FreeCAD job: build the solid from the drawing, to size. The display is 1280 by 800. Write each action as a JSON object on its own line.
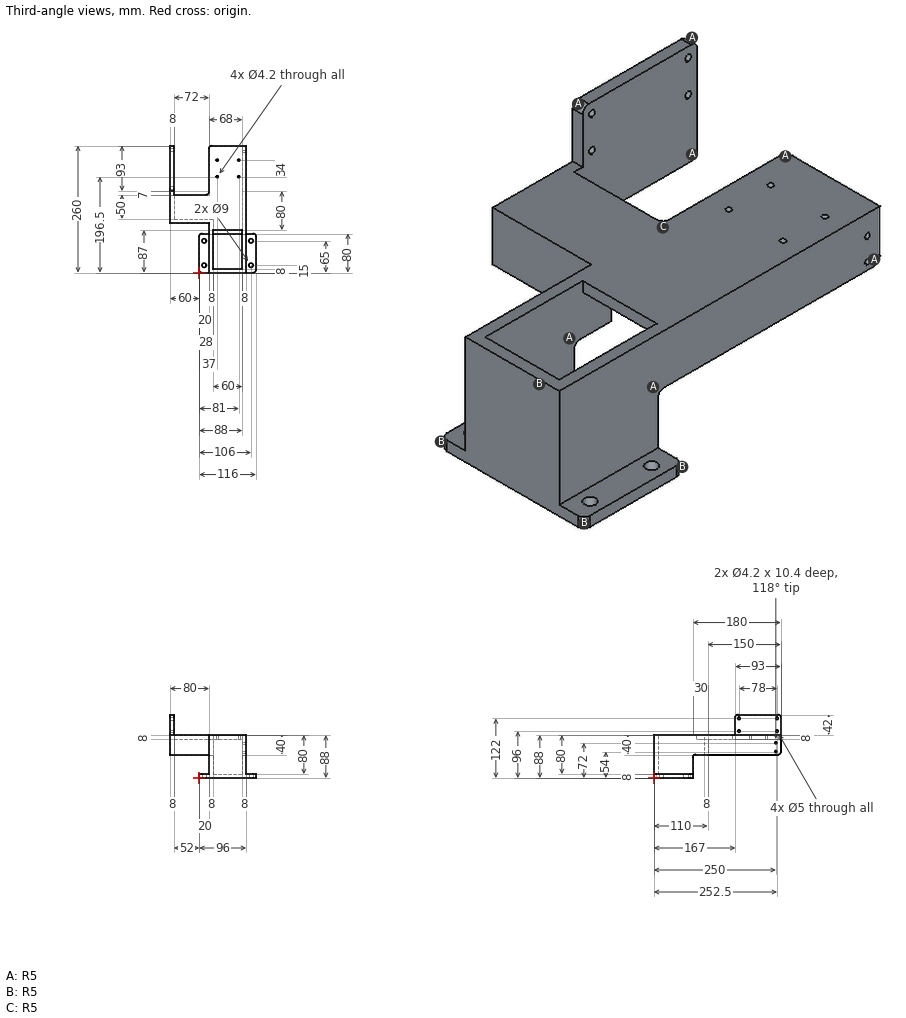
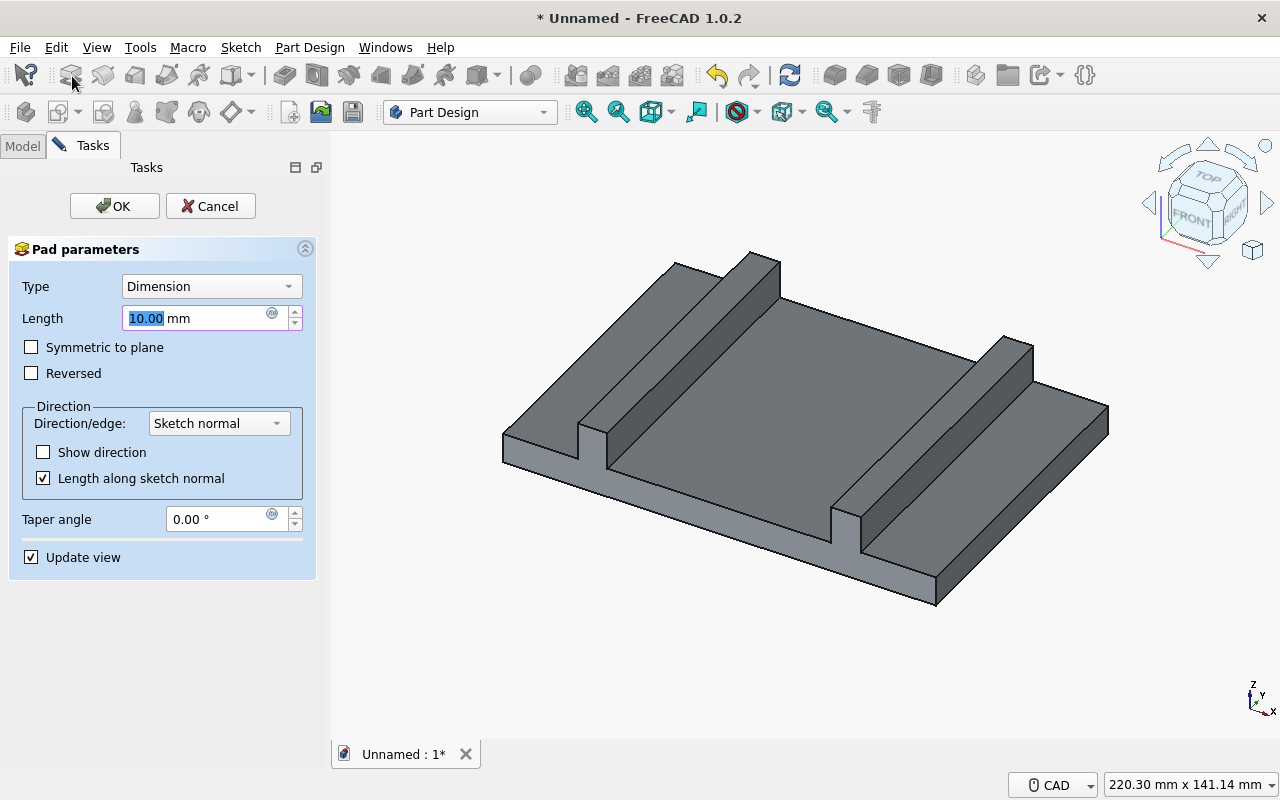
{"action": "type", "text": "80"}
{"action": "key", "text": "Tab"}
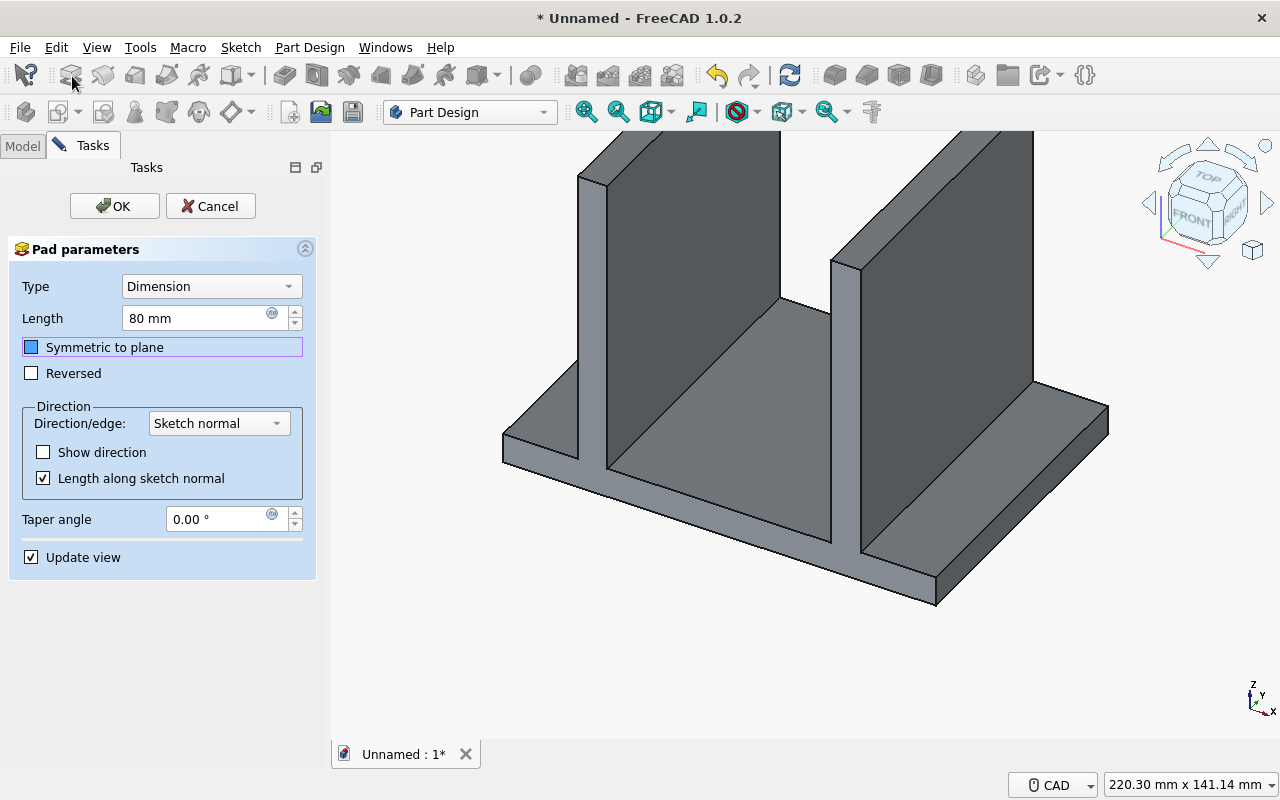
{"action": "left_click", "coordinate": [115, 206]}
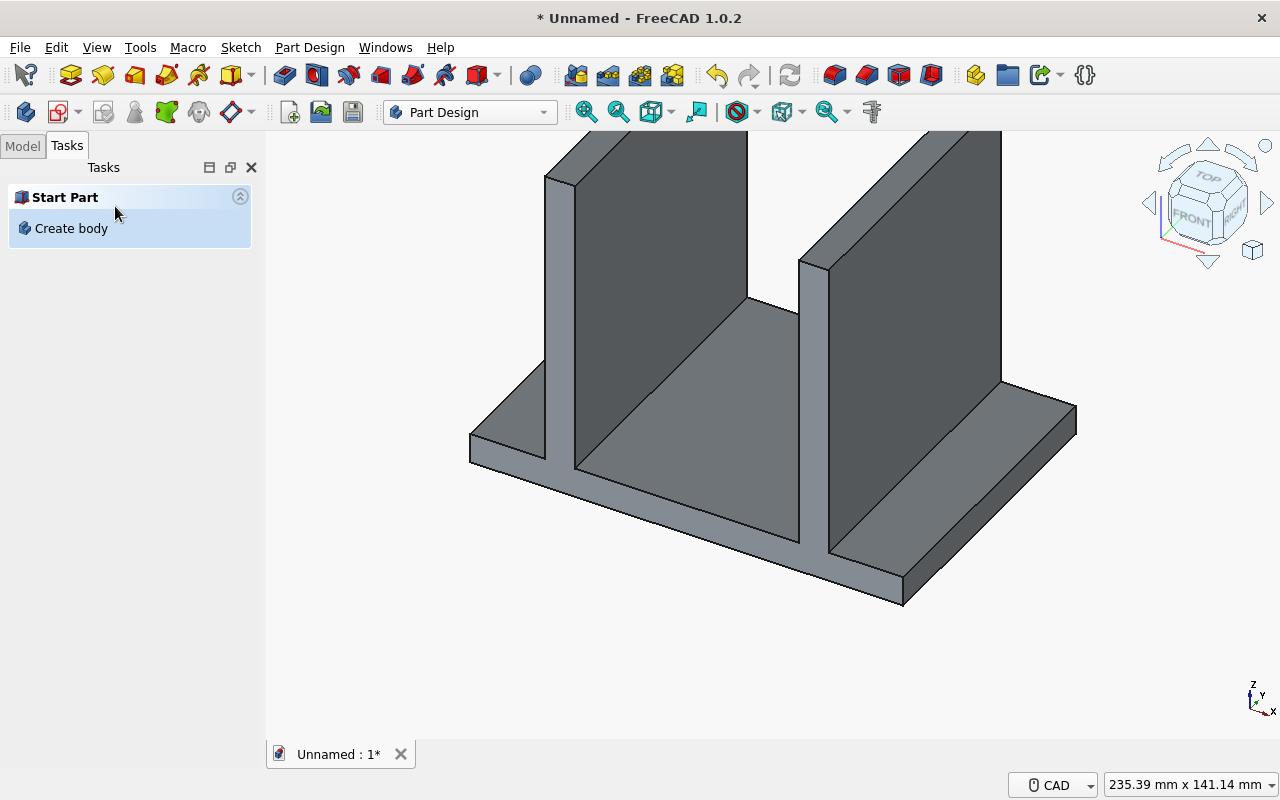
{"action": "left_click", "coordinate": [588, 112]}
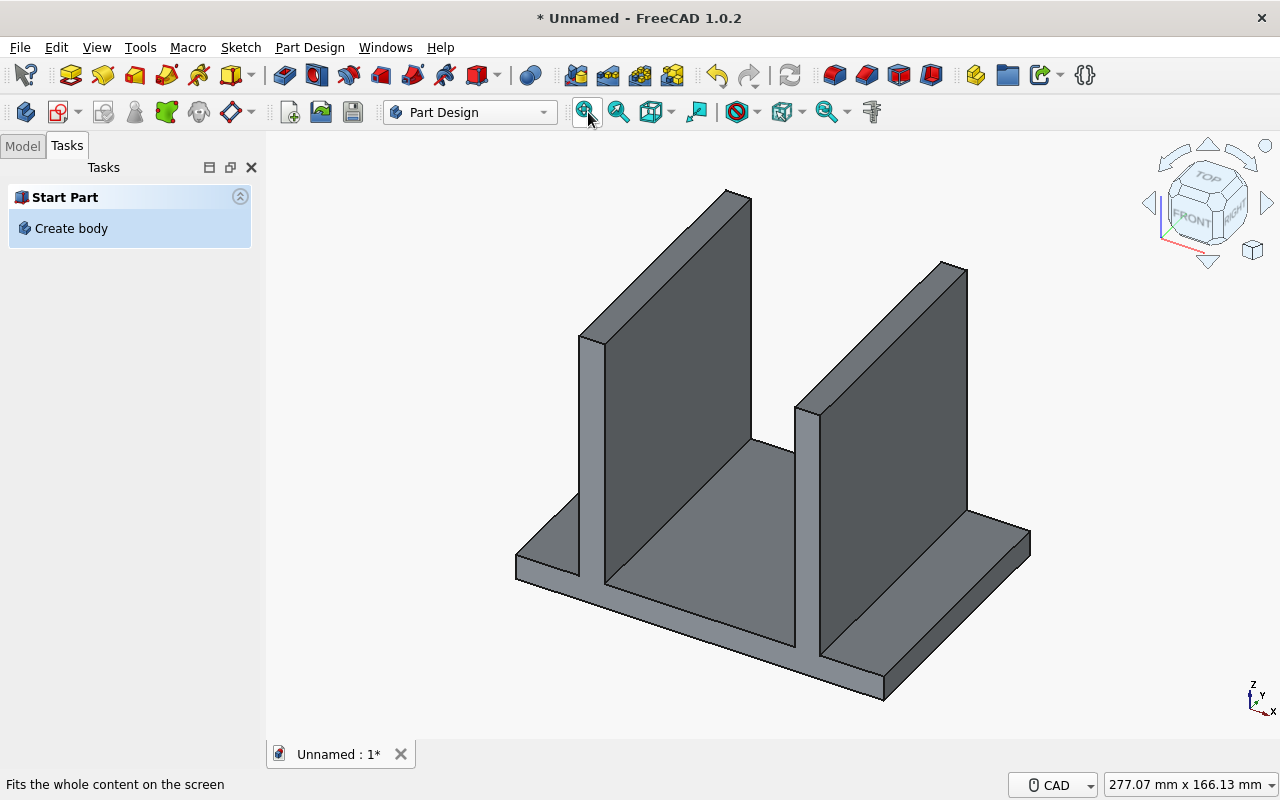
{"action": "key", "text": "4"}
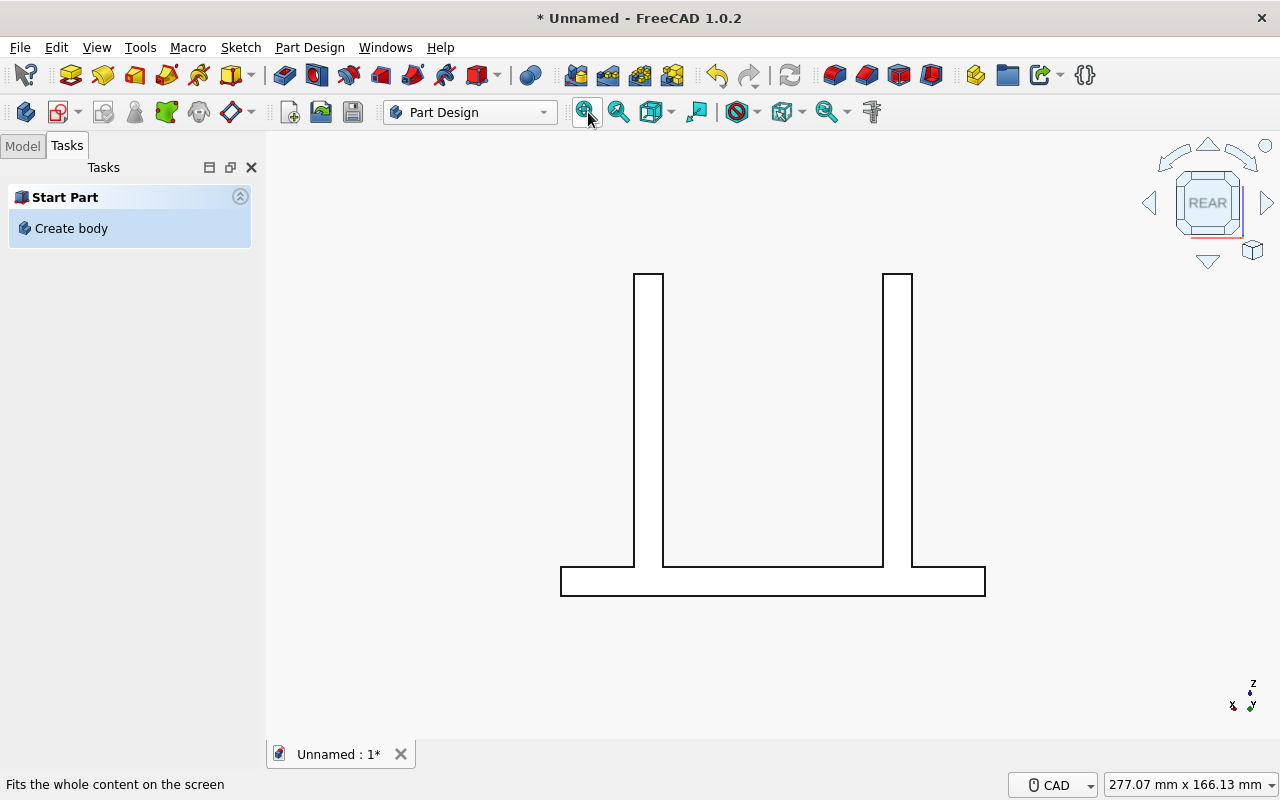
{"action": "left_click", "coordinate": [652, 572]}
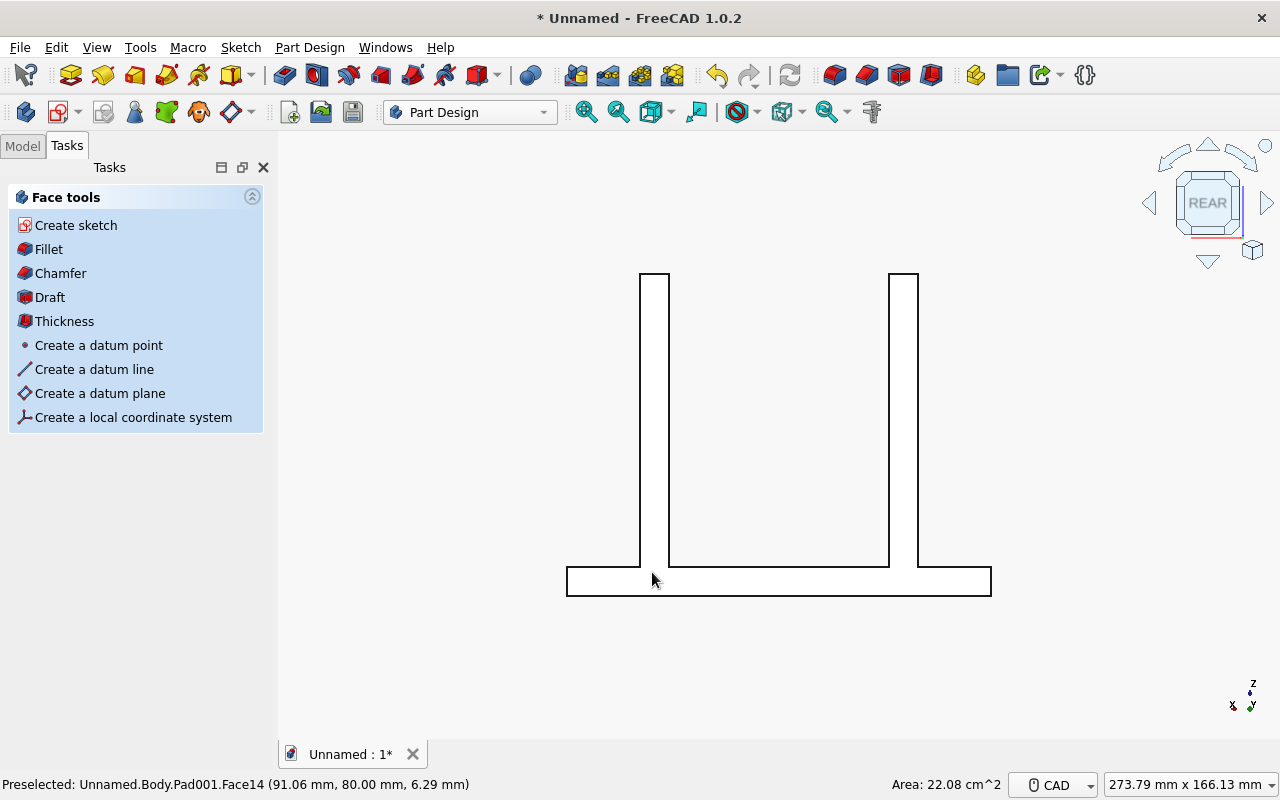
{"action": "left_click", "coordinate": [58, 112]}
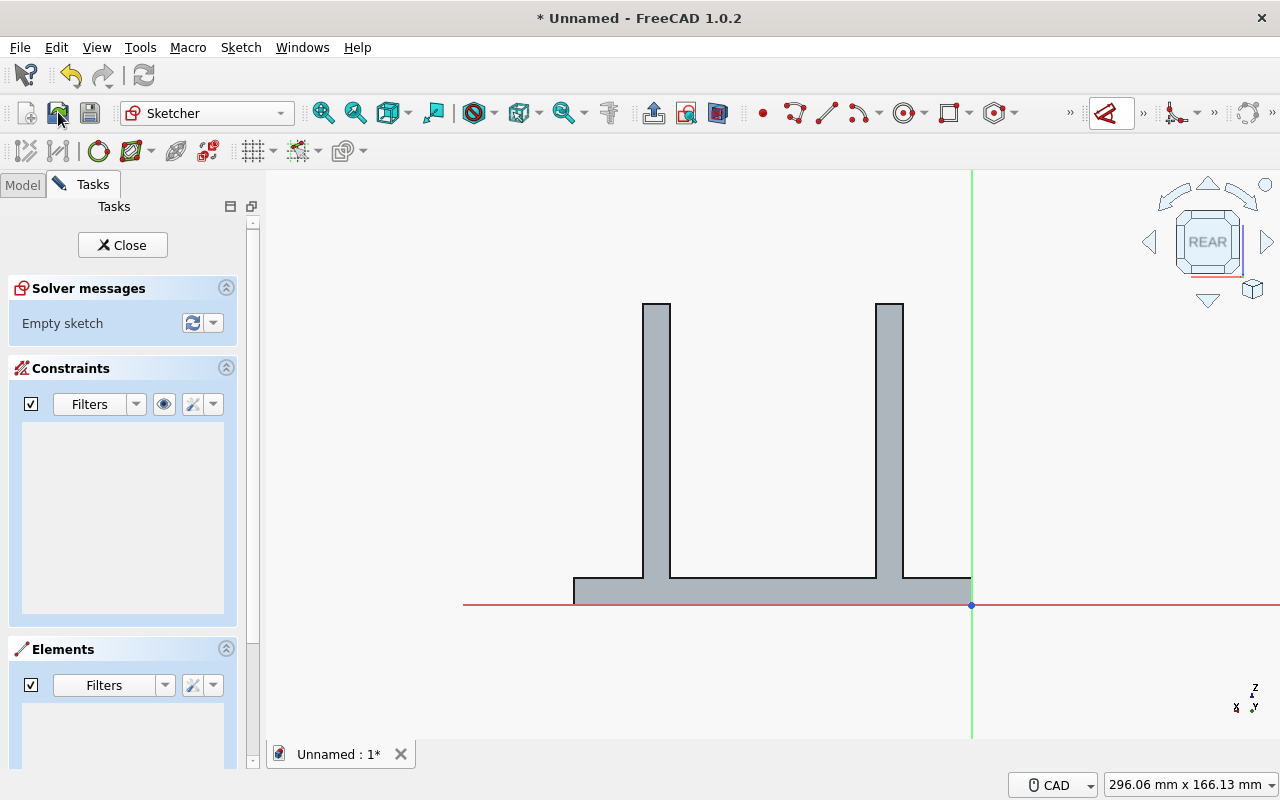
{"action": "left_click", "coordinate": [950, 114]}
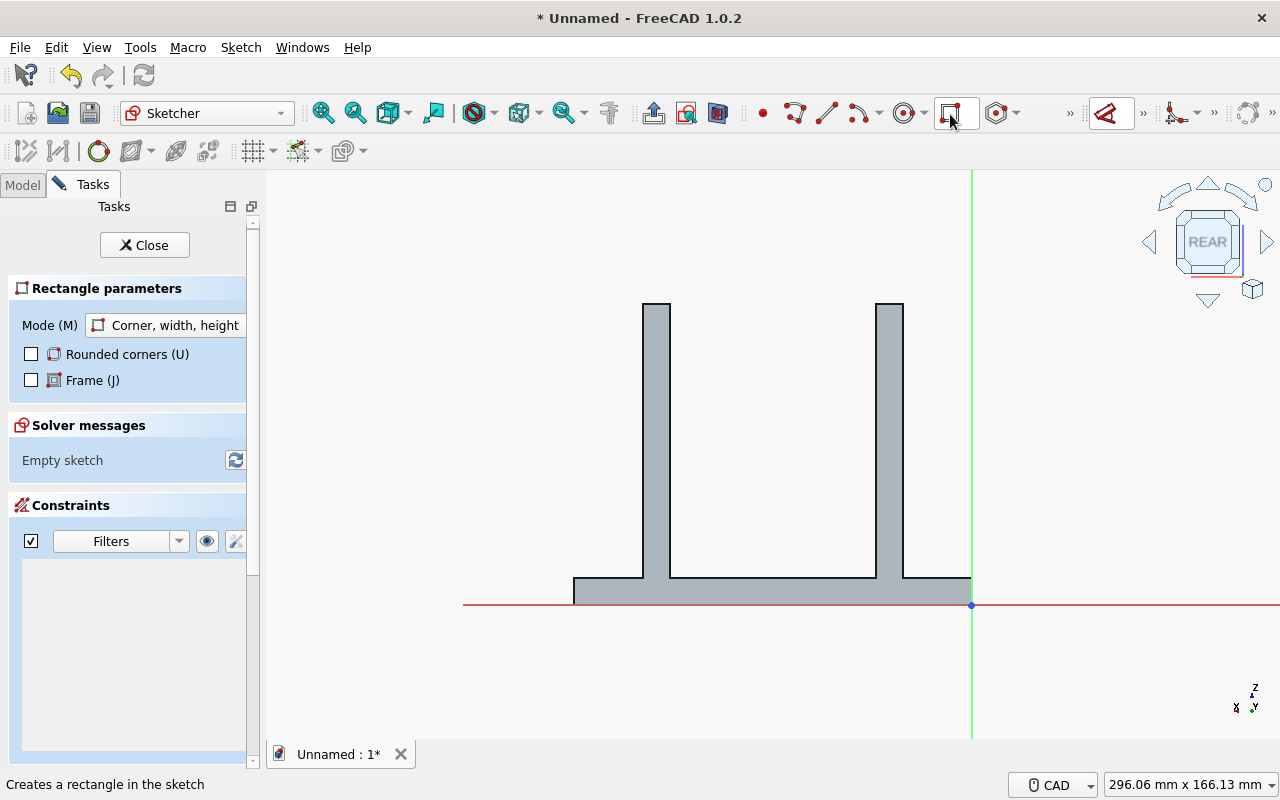
{"action": "left_click", "coordinate": [643, 304]}
{"action": "left_click", "coordinate": [670, 441]}
{"action": "key", "text": "Escape"}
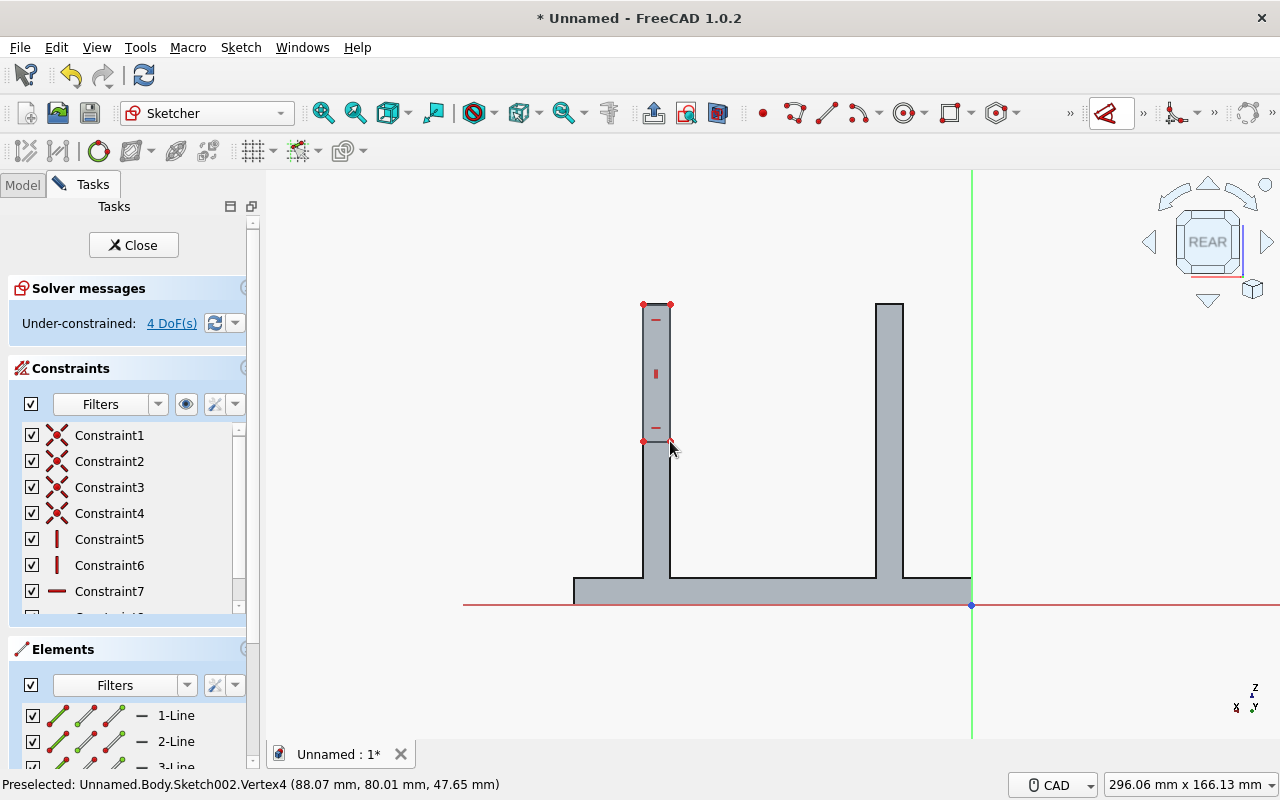
{"action": "scroll", "coordinate": [654, 442], "scroll_direction": "up", "scroll_amount": 2}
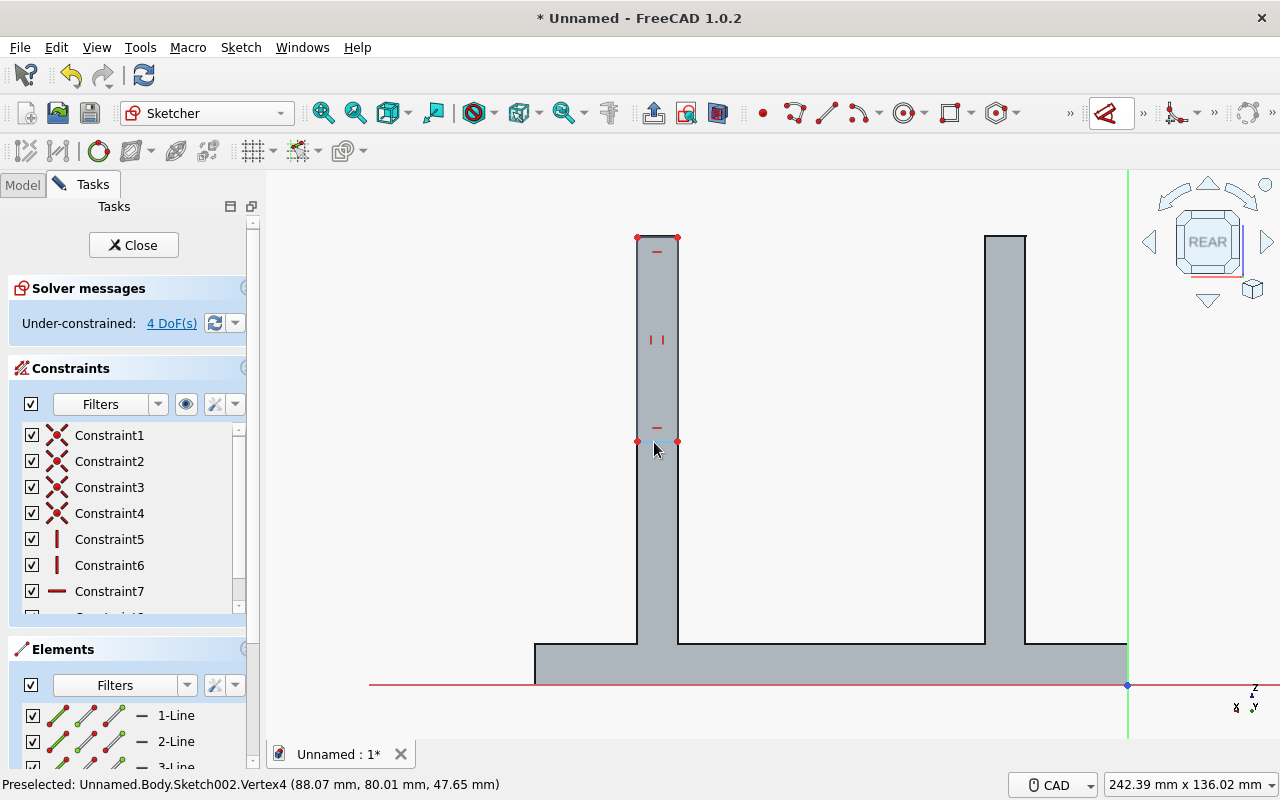
{"action": "left_click", "coordinate": [654, 442]}